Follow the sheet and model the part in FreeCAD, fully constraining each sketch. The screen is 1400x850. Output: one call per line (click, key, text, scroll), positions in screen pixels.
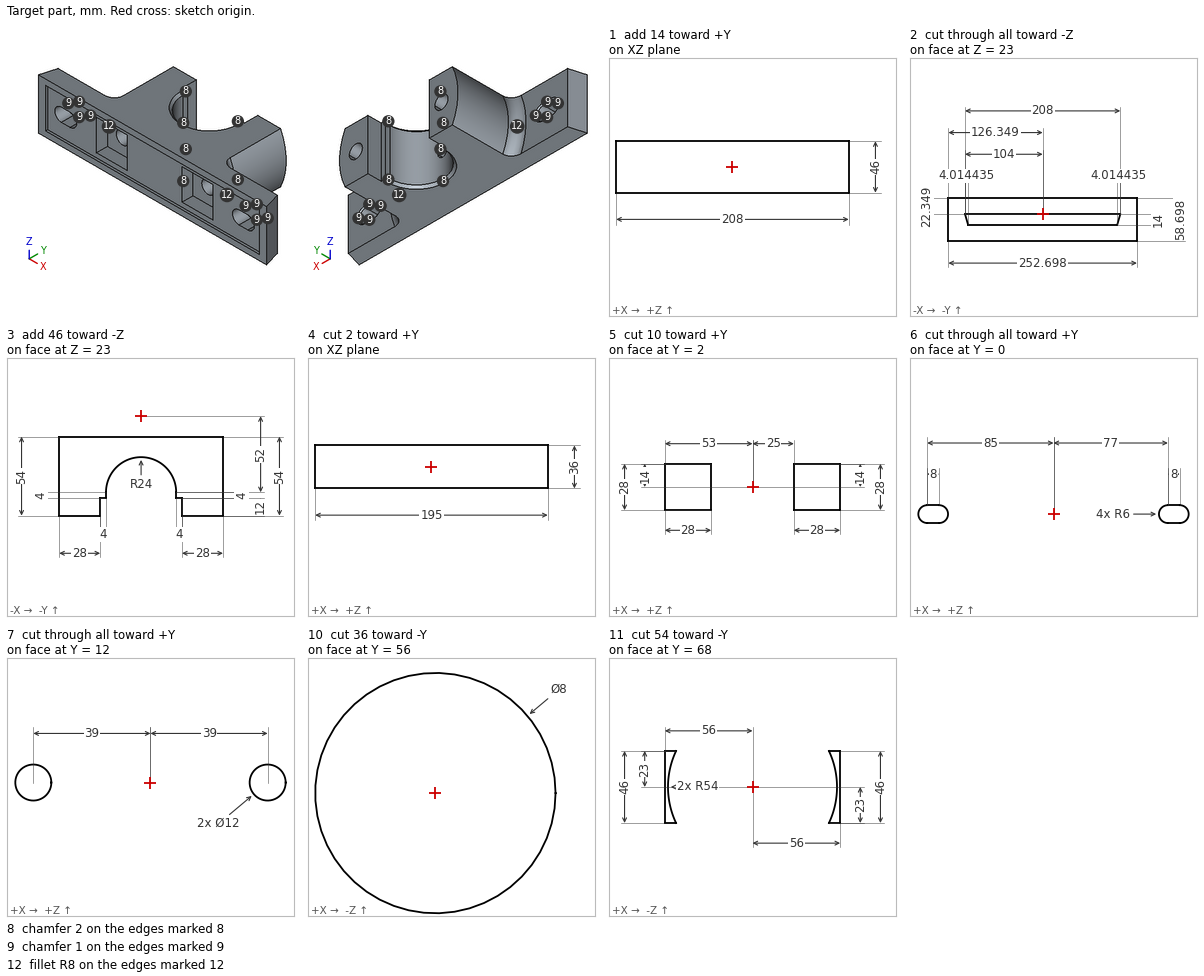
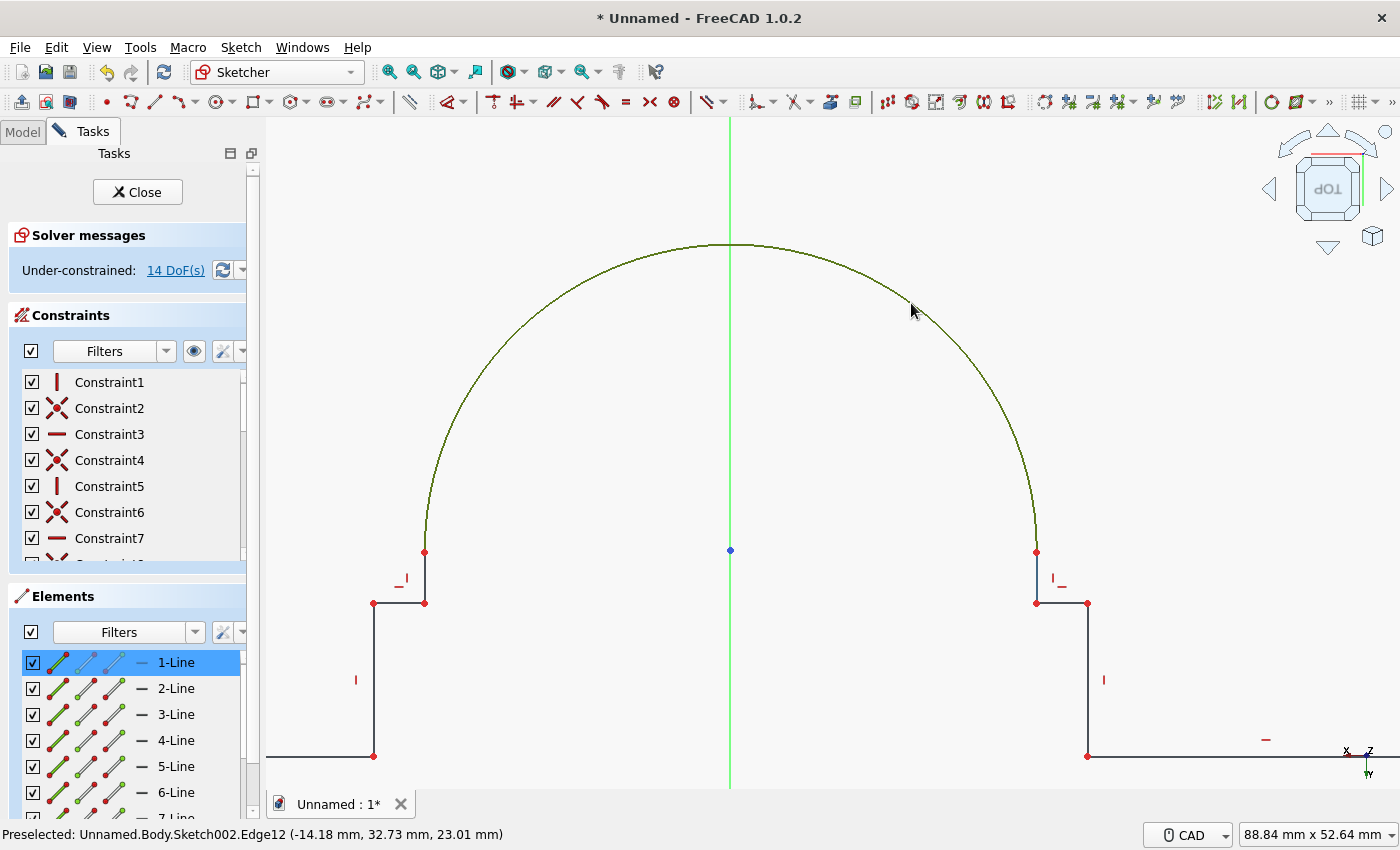
click(602, 102)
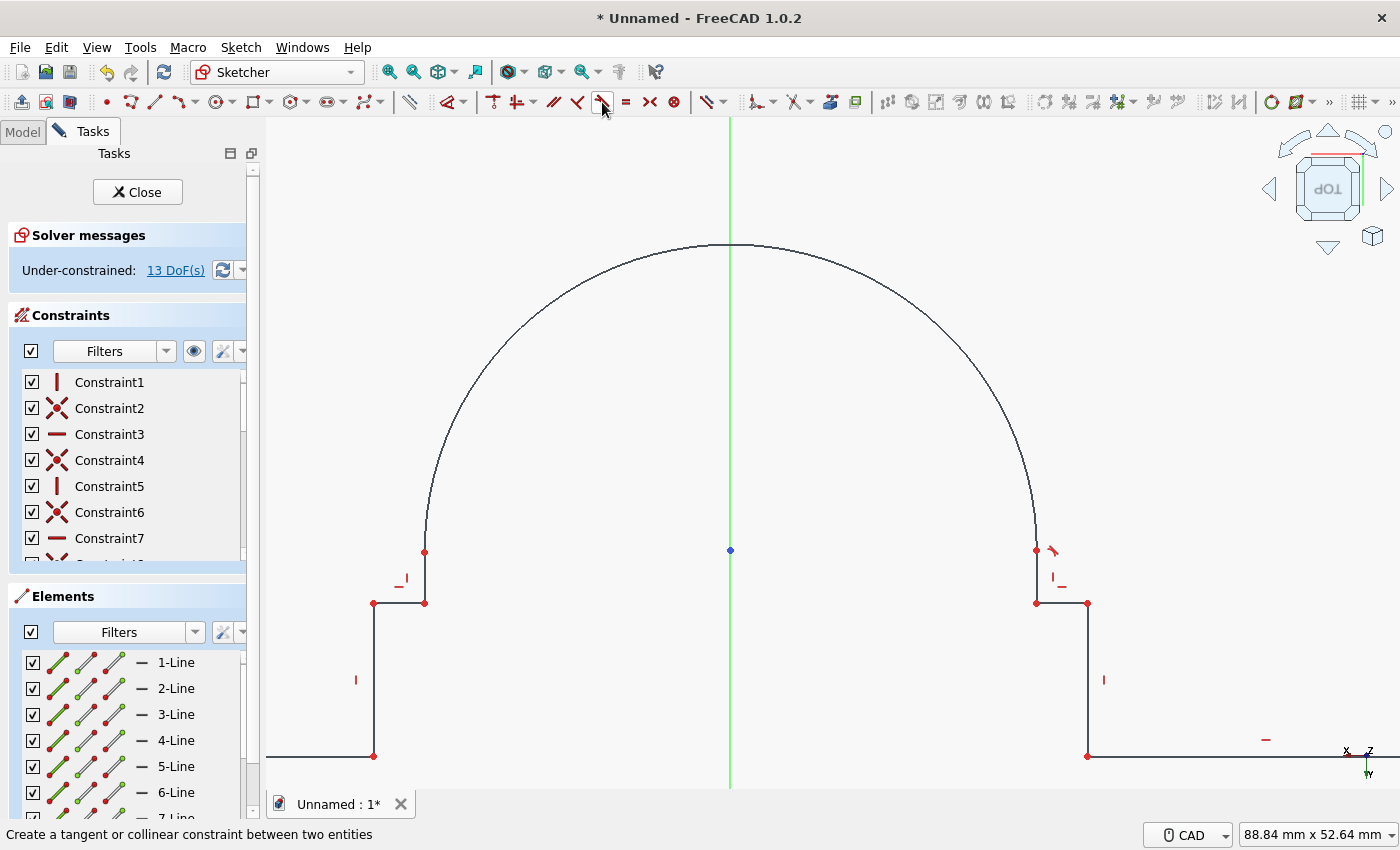
click(425, 588)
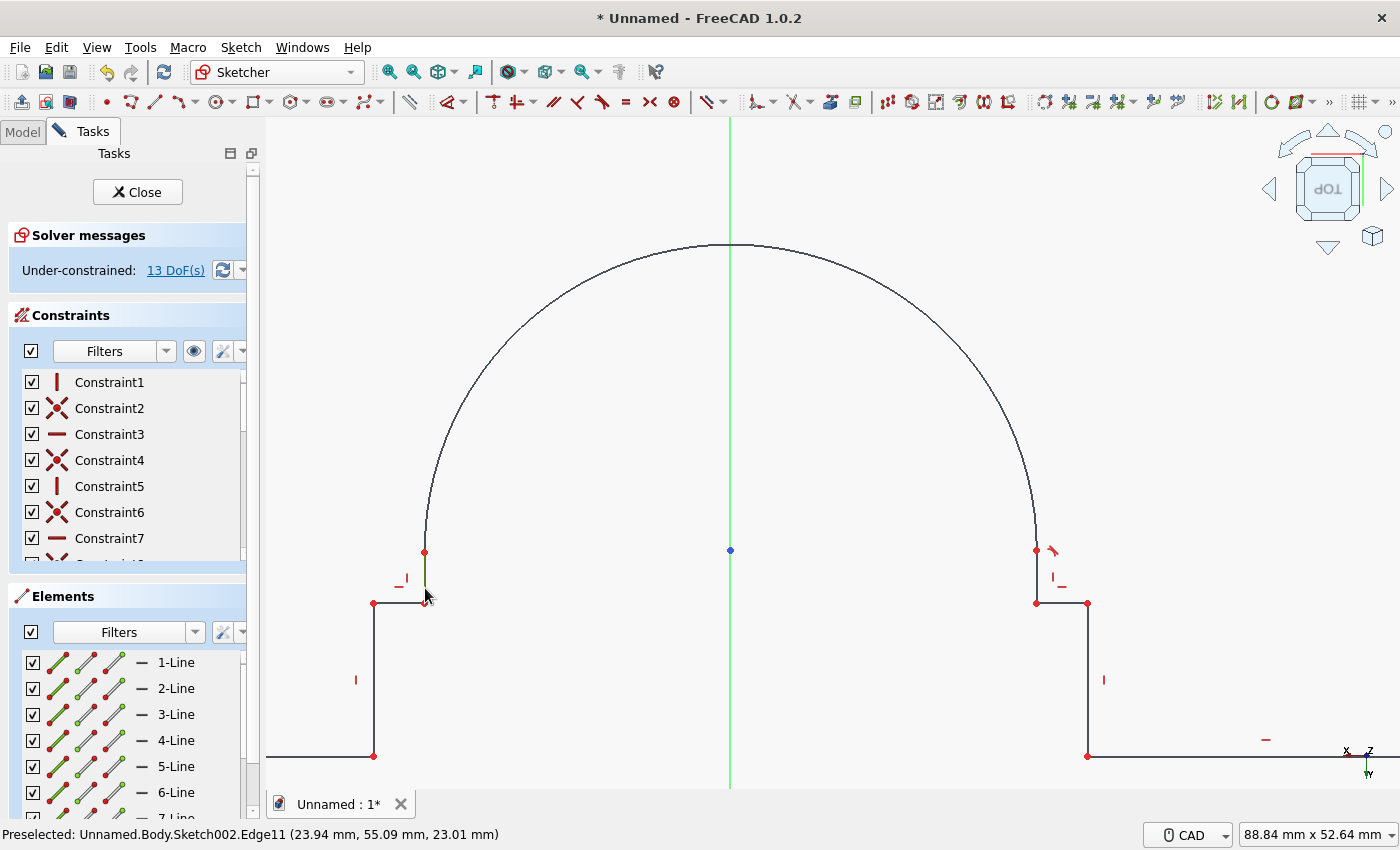
click(910, 303)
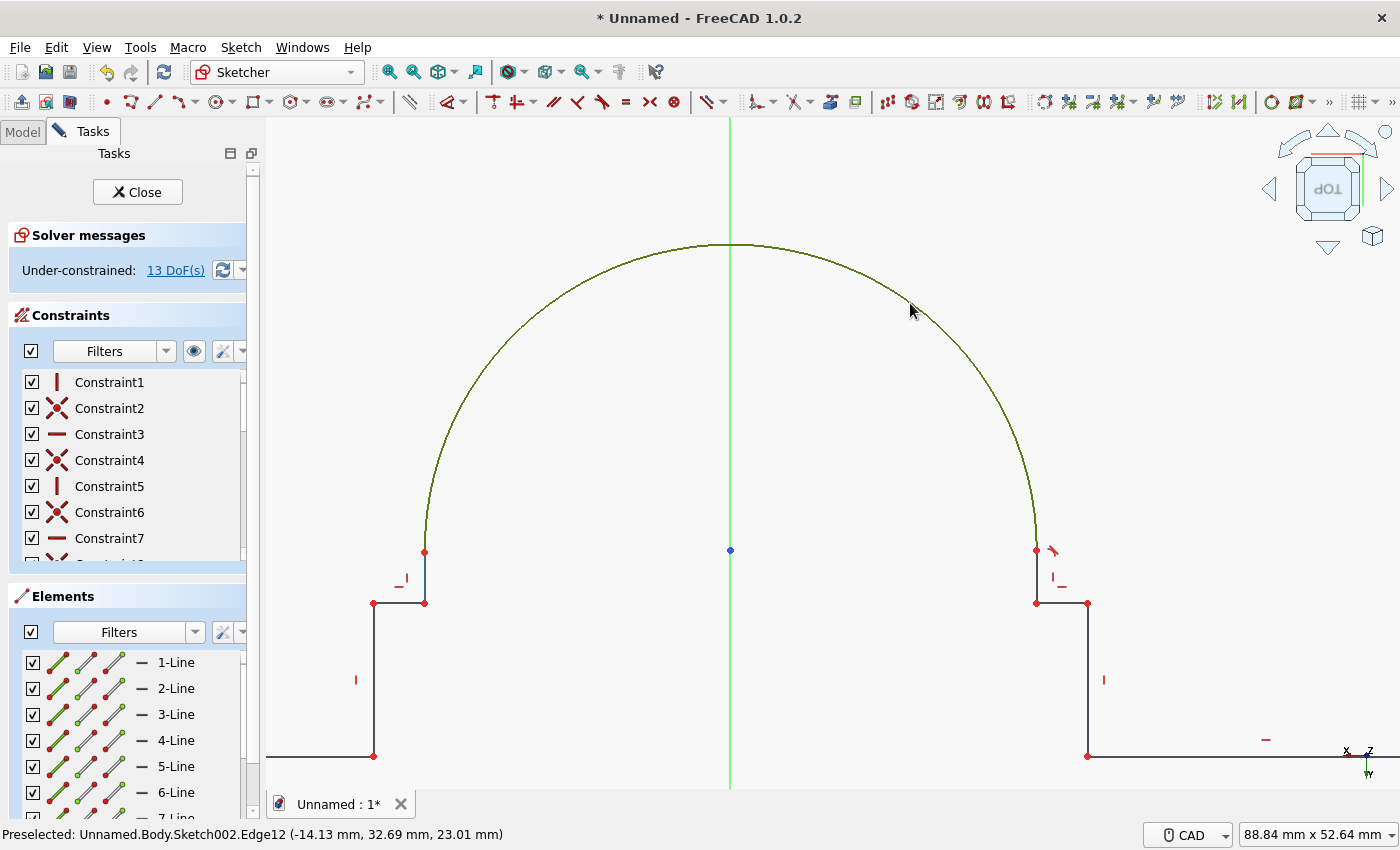
key(t)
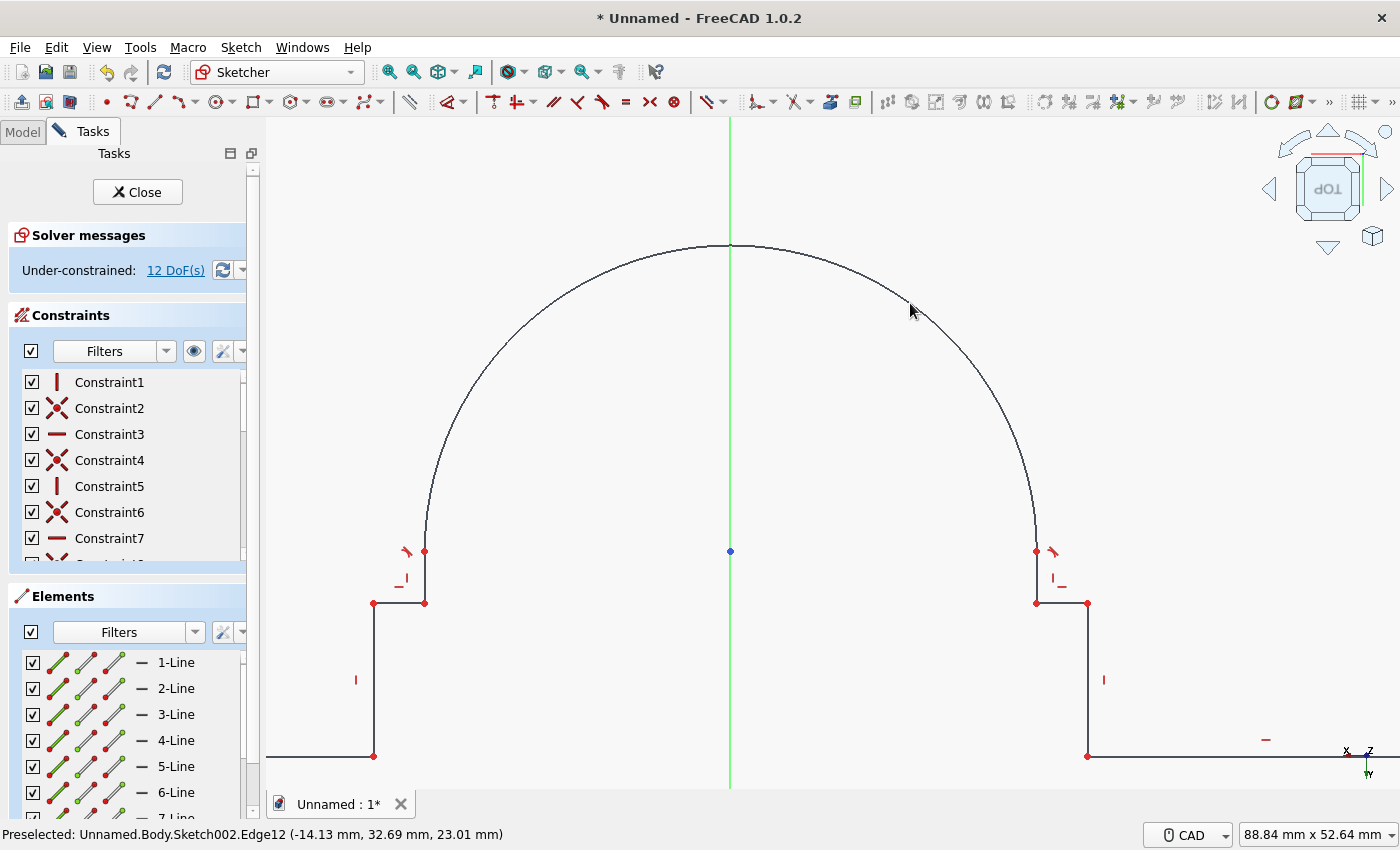
click(731, 551)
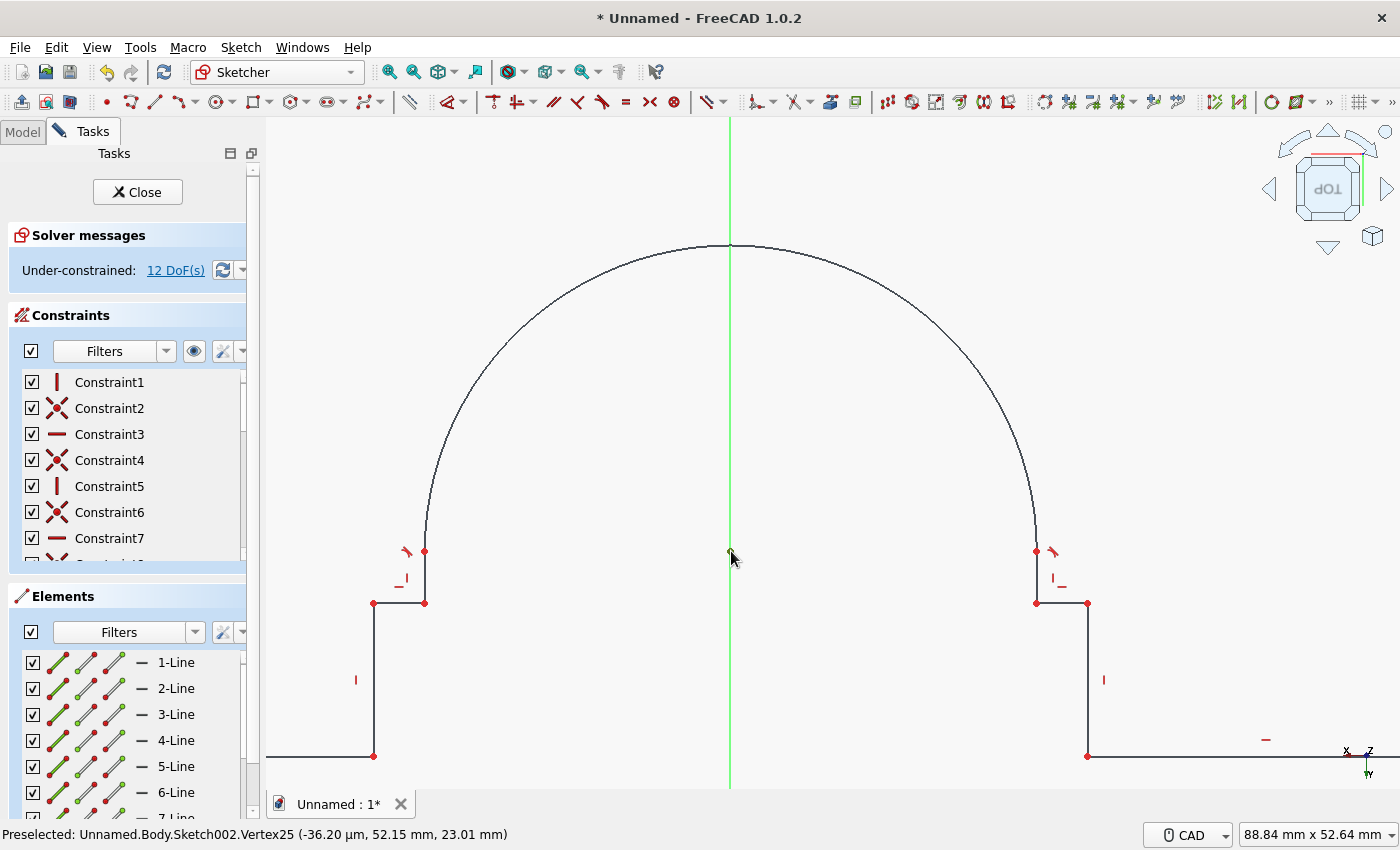
click(730, 717)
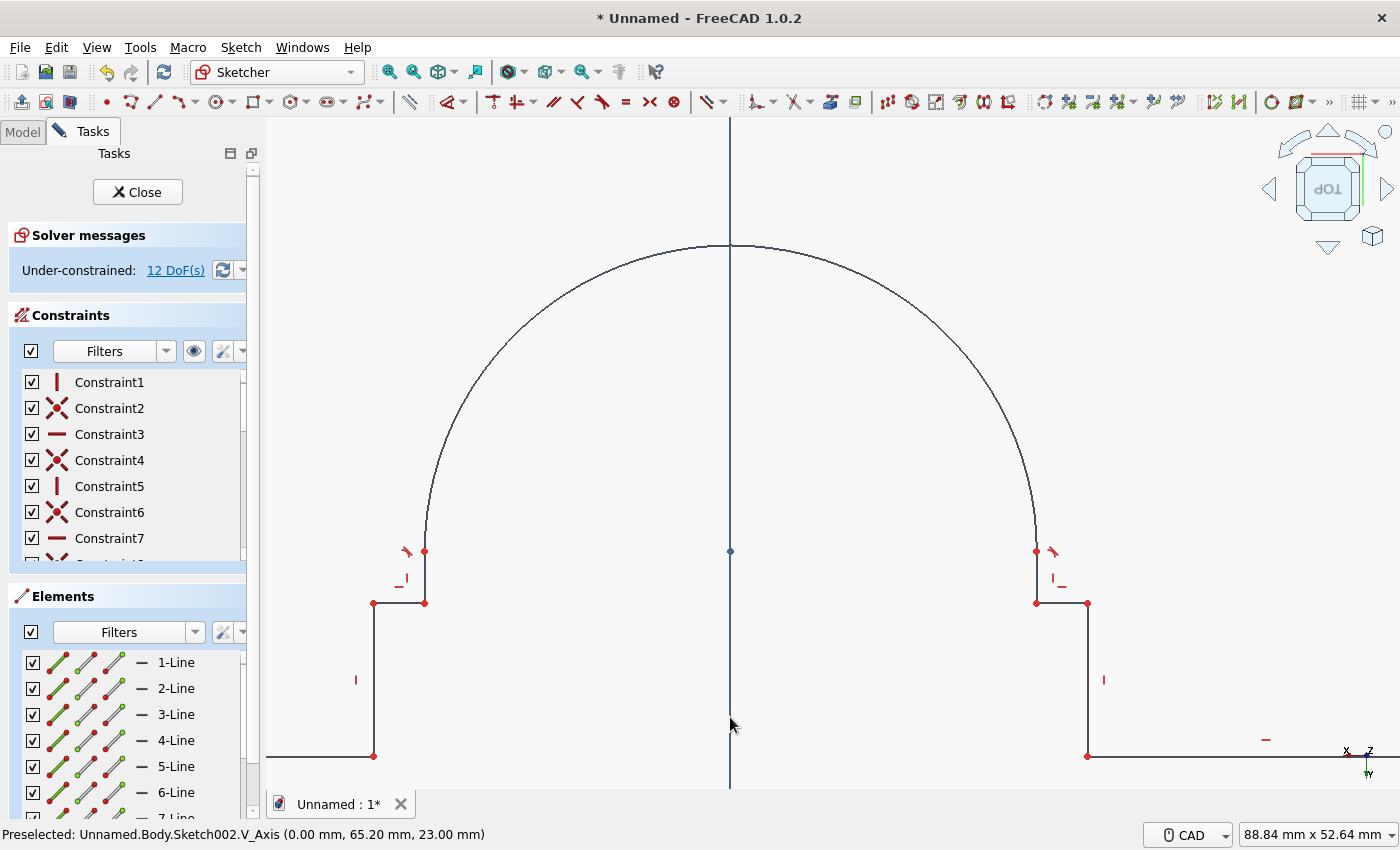
click(494, 102)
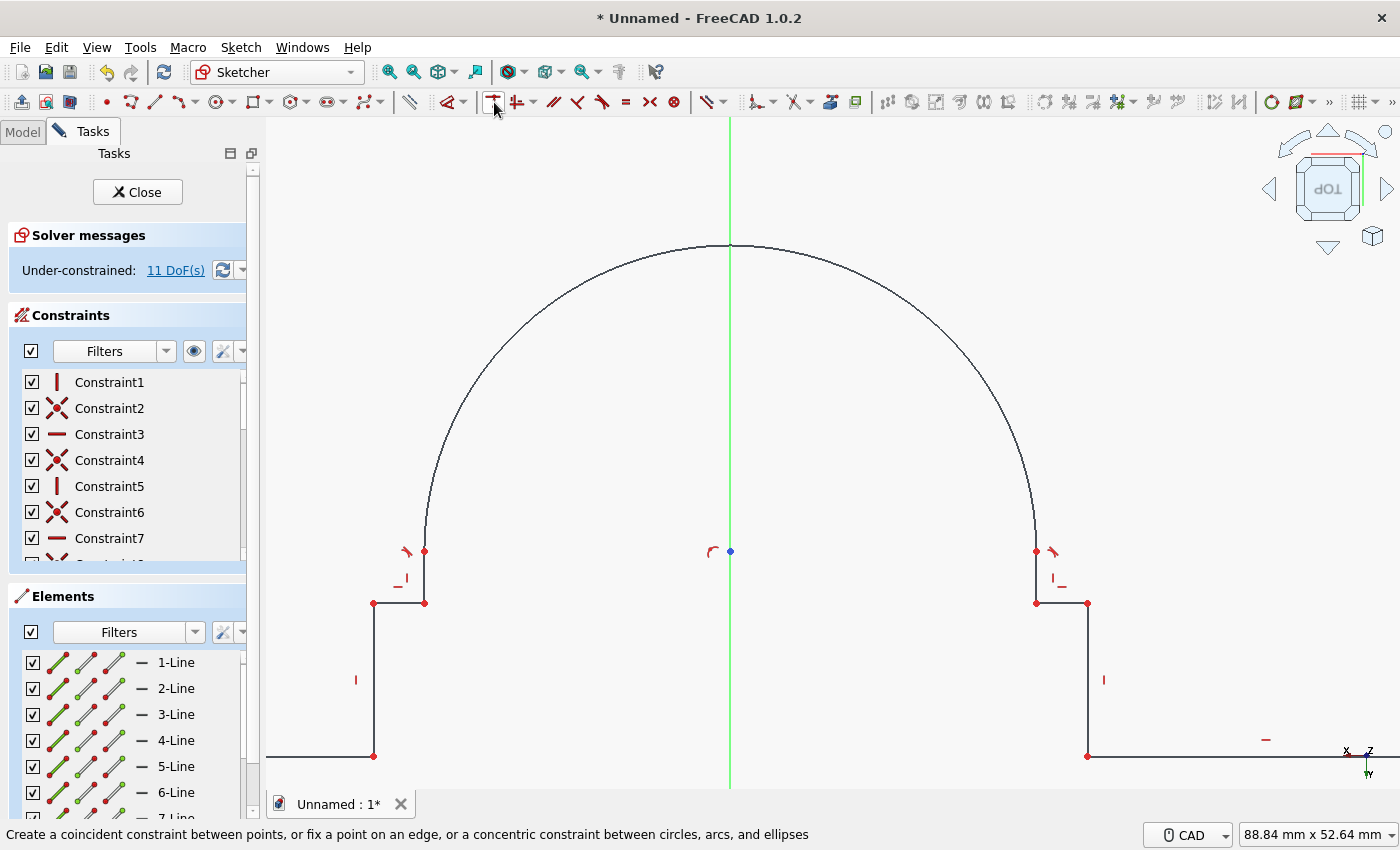
key(d)